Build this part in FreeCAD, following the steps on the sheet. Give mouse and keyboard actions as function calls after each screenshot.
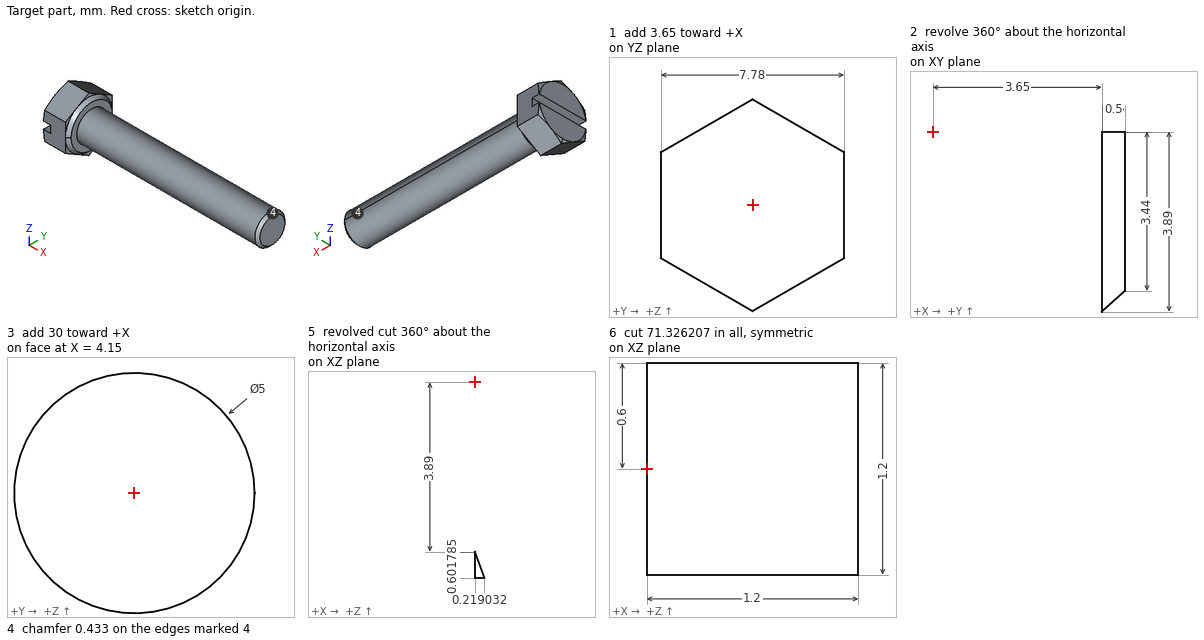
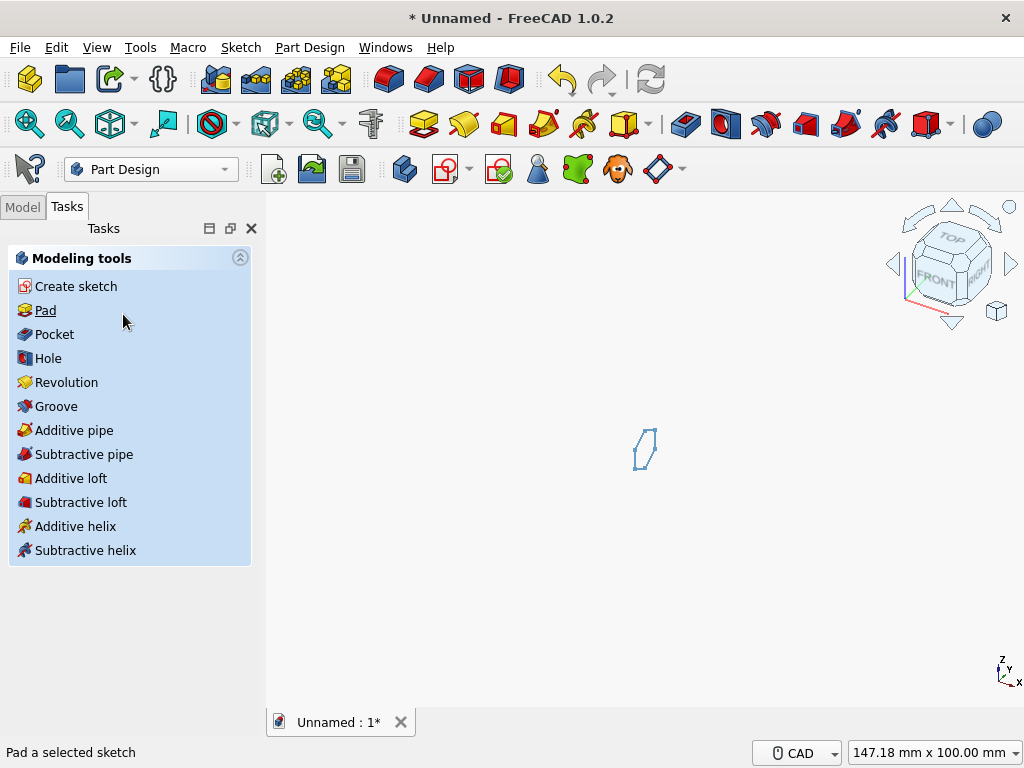
click(424, 124)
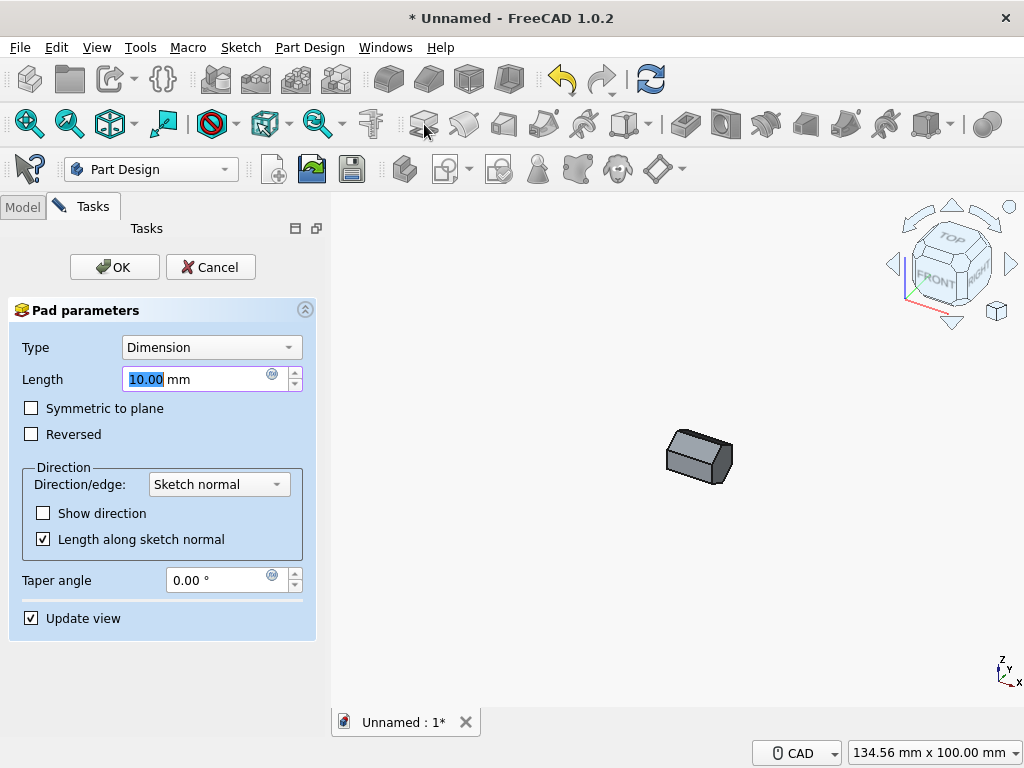
text(3.65)
key(Tab)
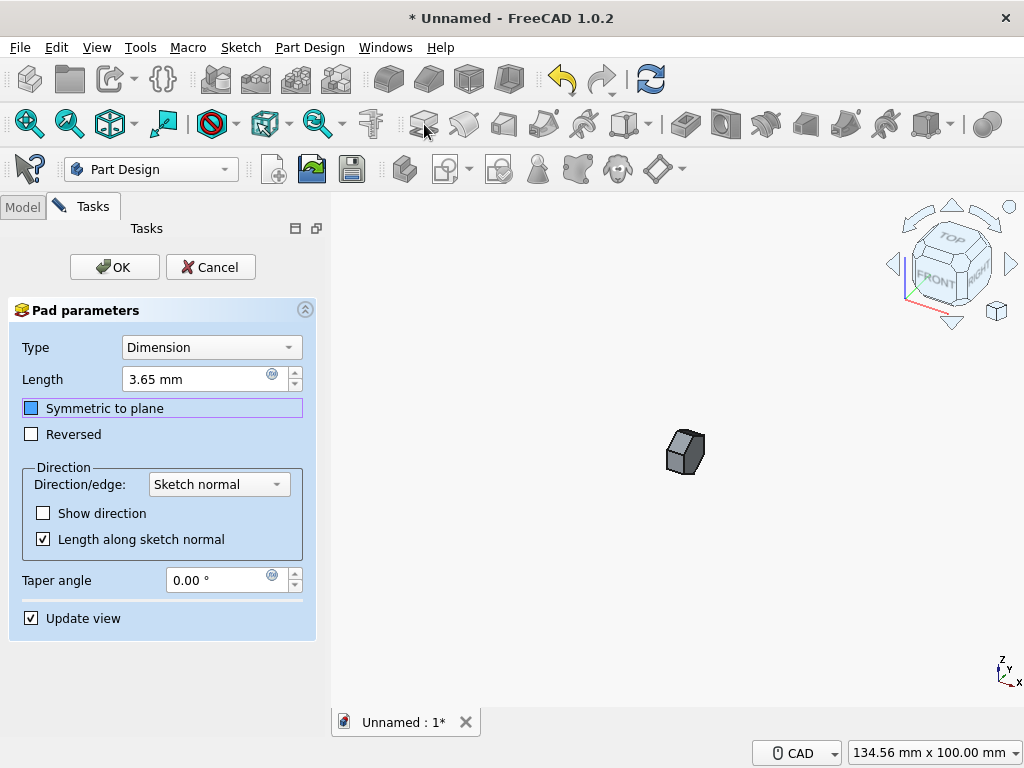
click(115, 267)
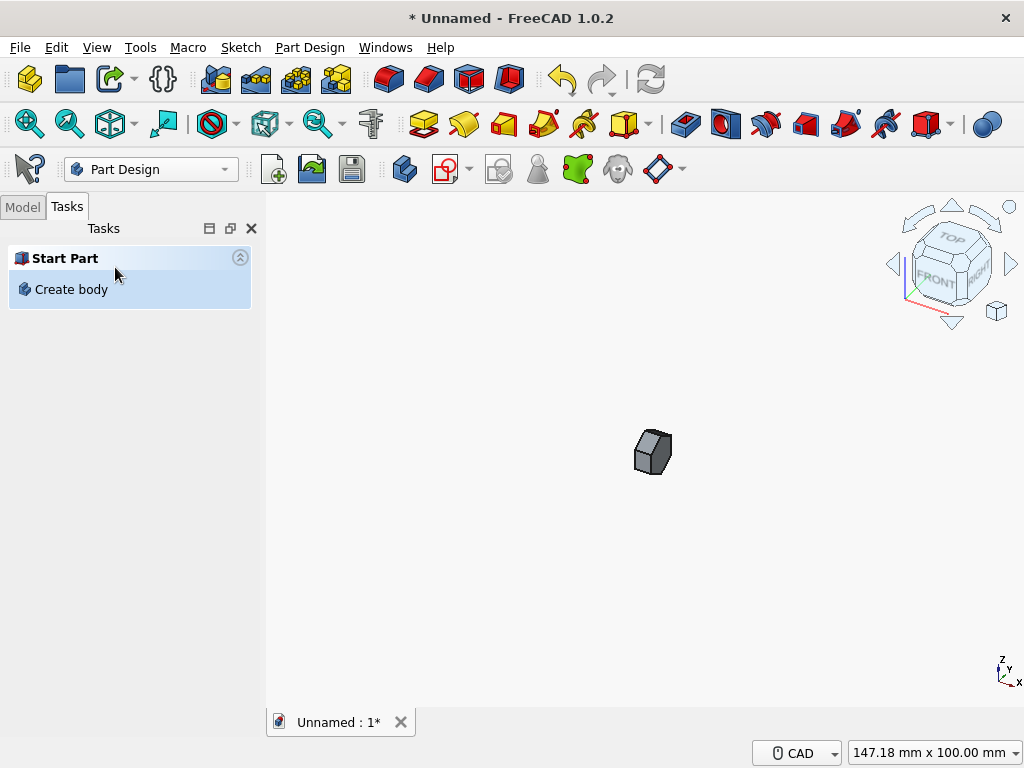
click(30, 124)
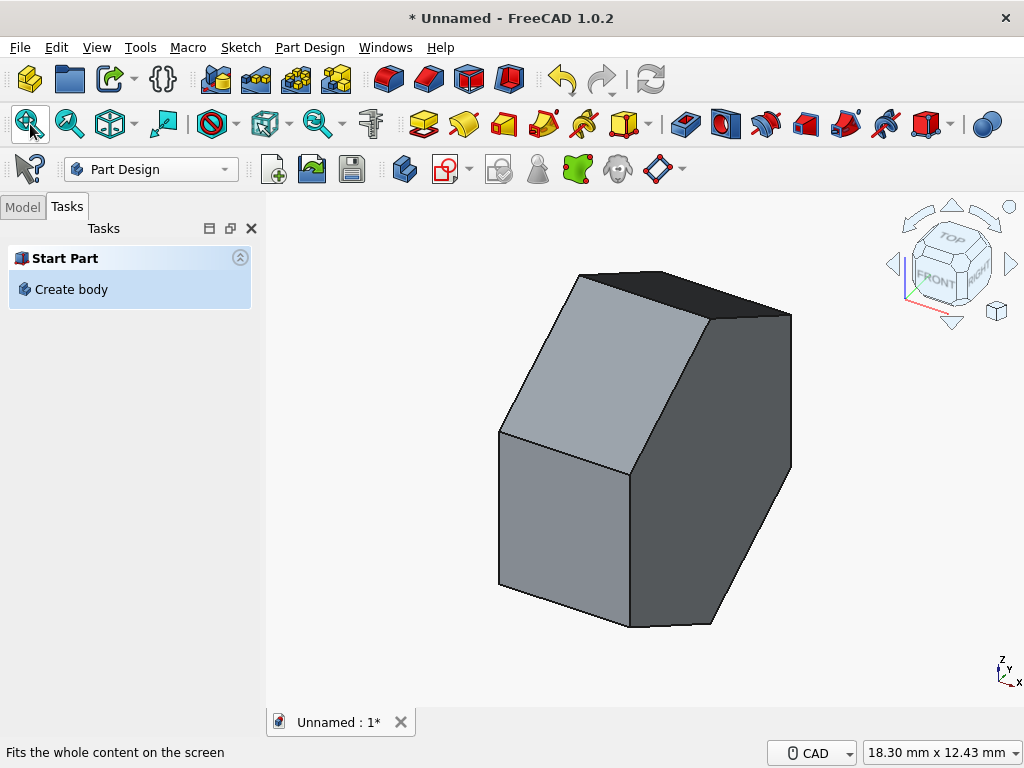
click(446, 170)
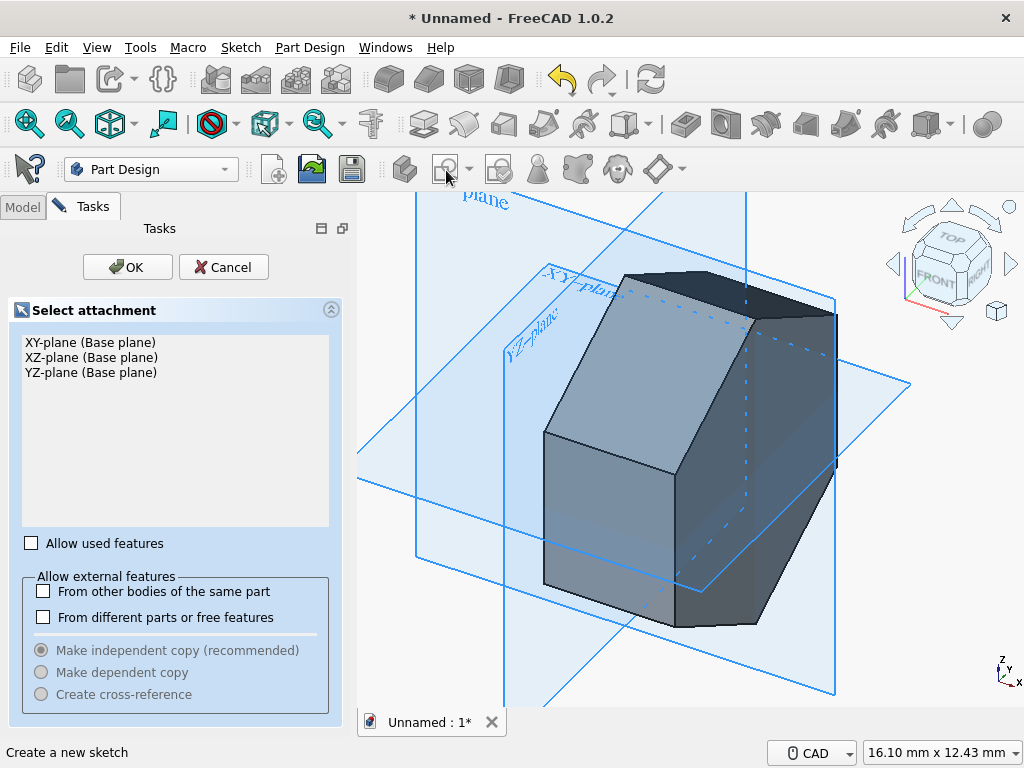
click(82, 342)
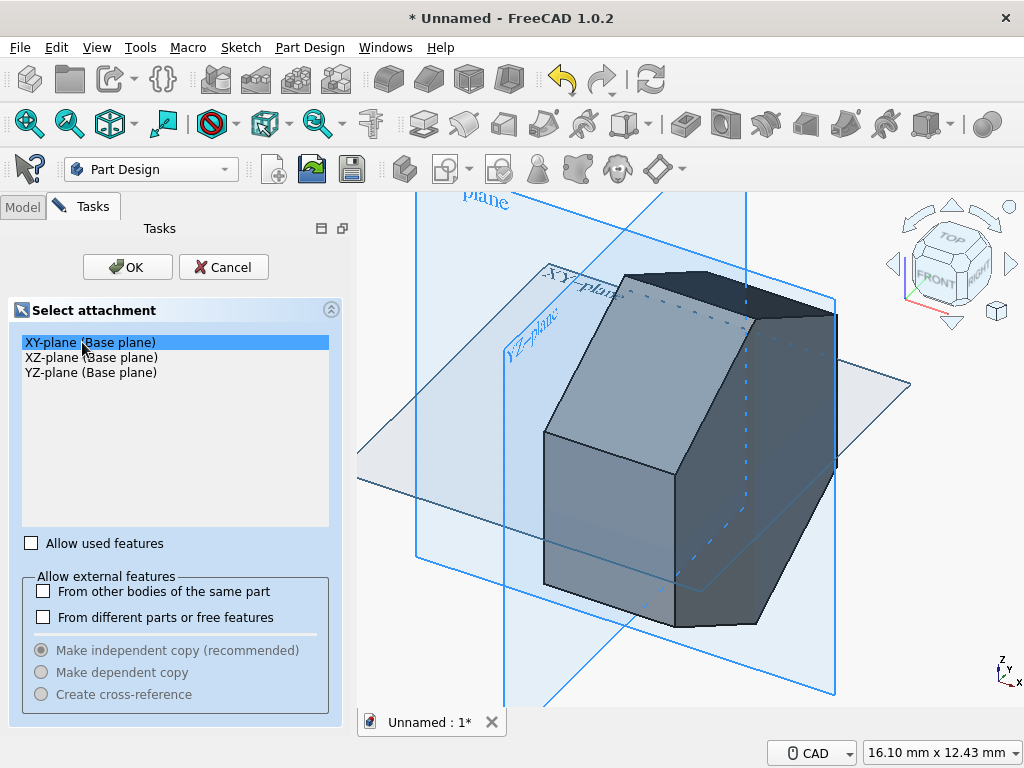
click(128, 267)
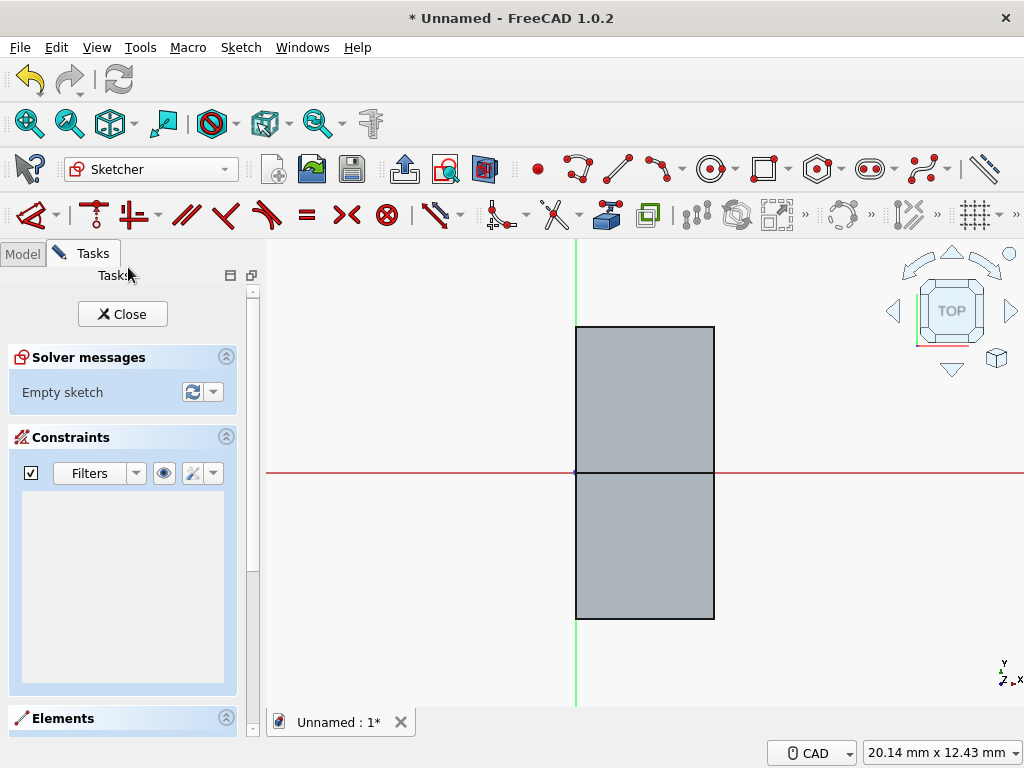
key(q)
key(s)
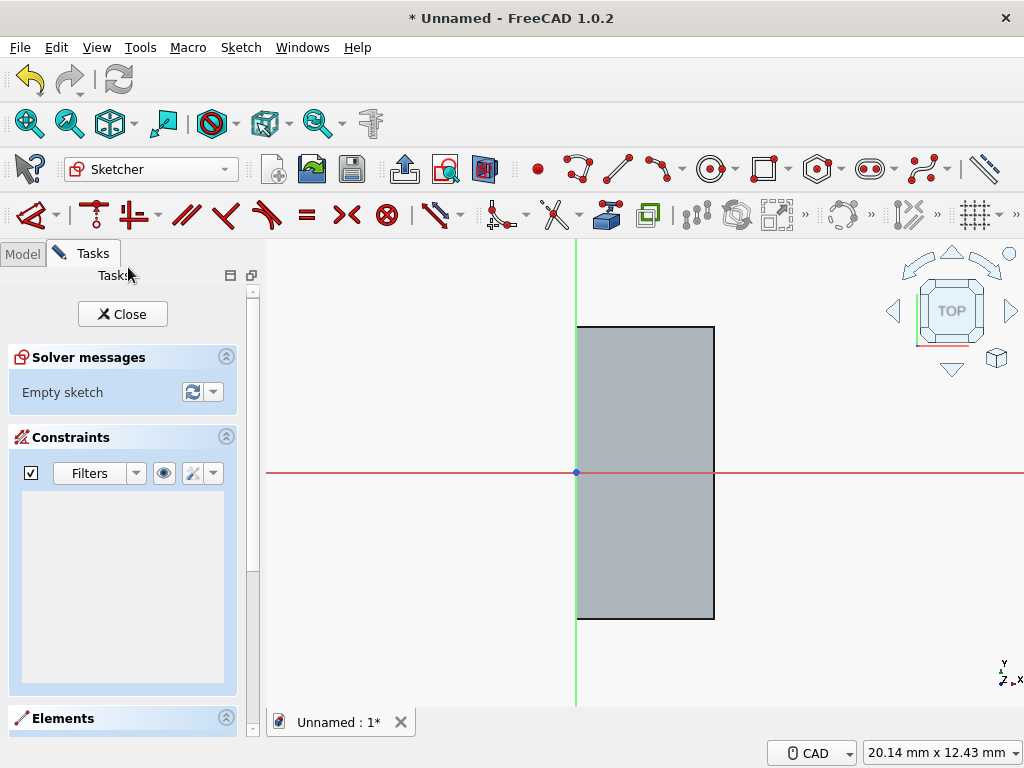
scroll(749, 635, up, 3)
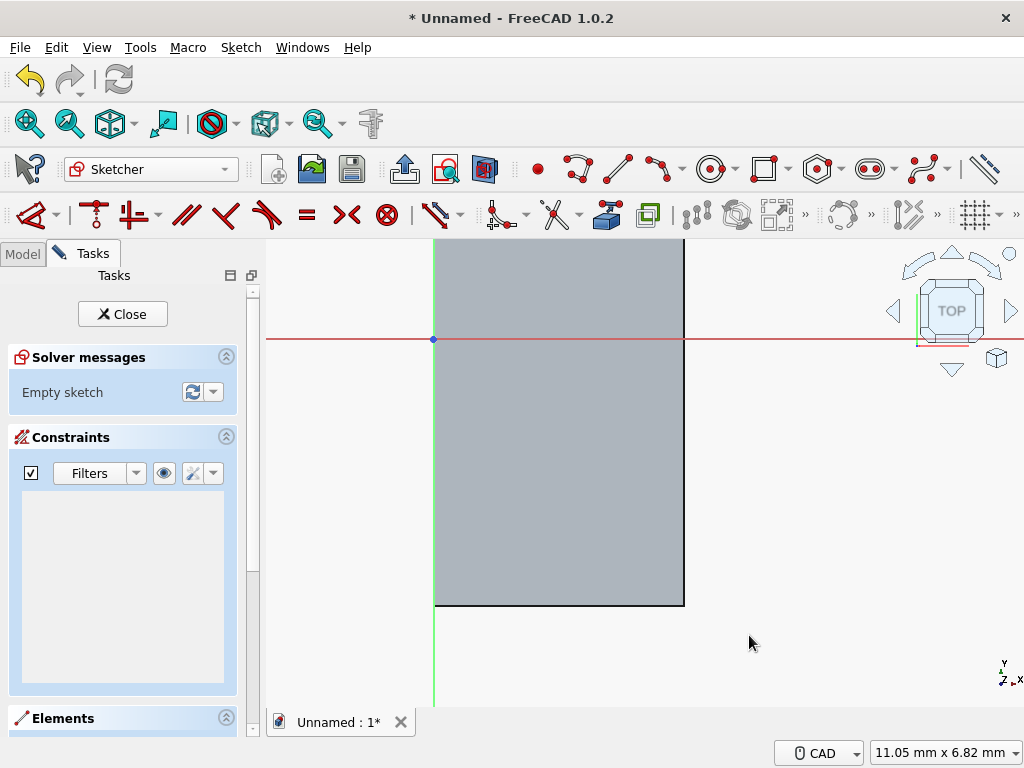
click(578, 170)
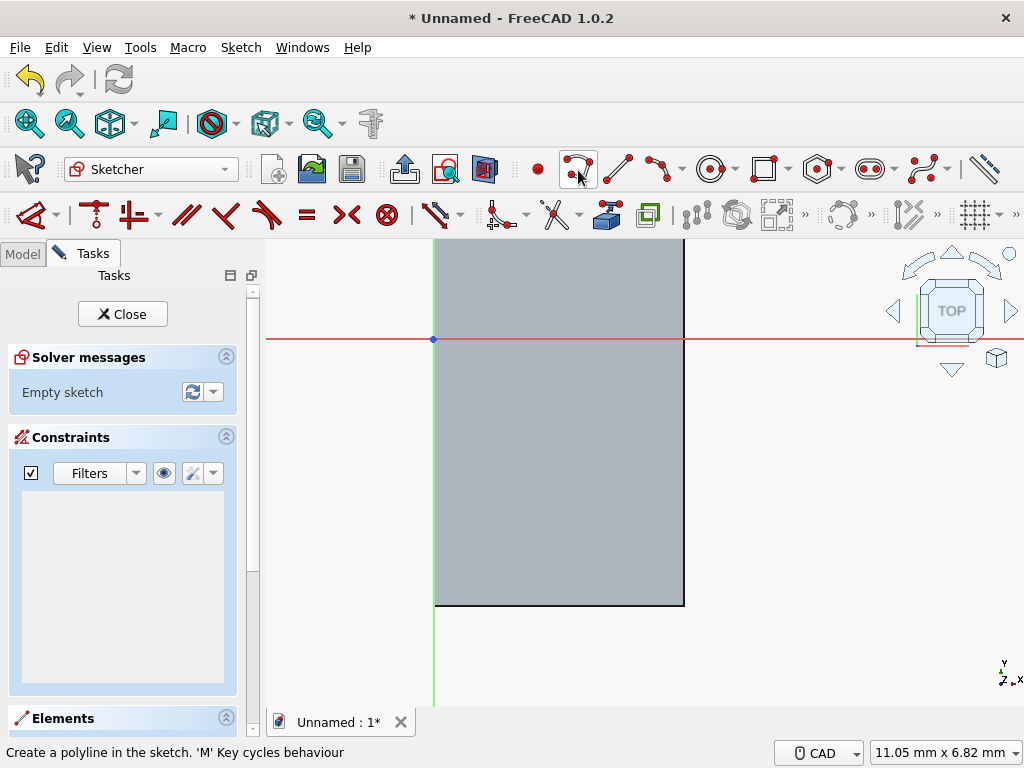
click(684, 339)
click(684, 606)
click(718, 575)
click(718, 348)
click(684, 339)
key(Escape)
key(Escape)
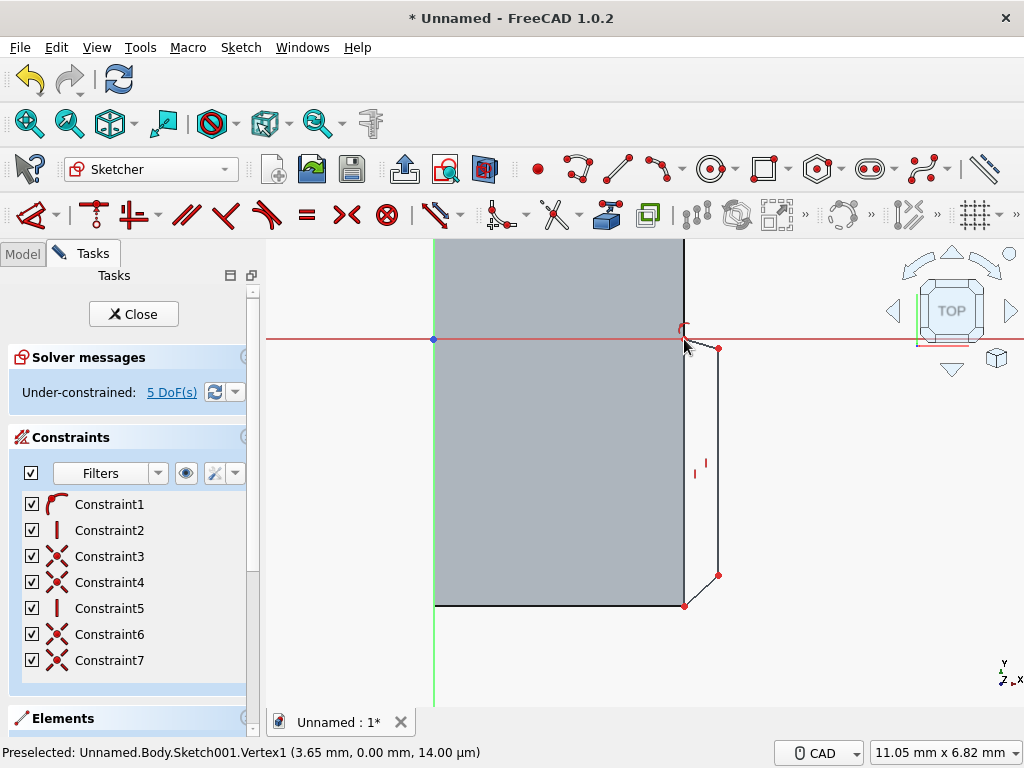
scroll(694, 342, up, 2)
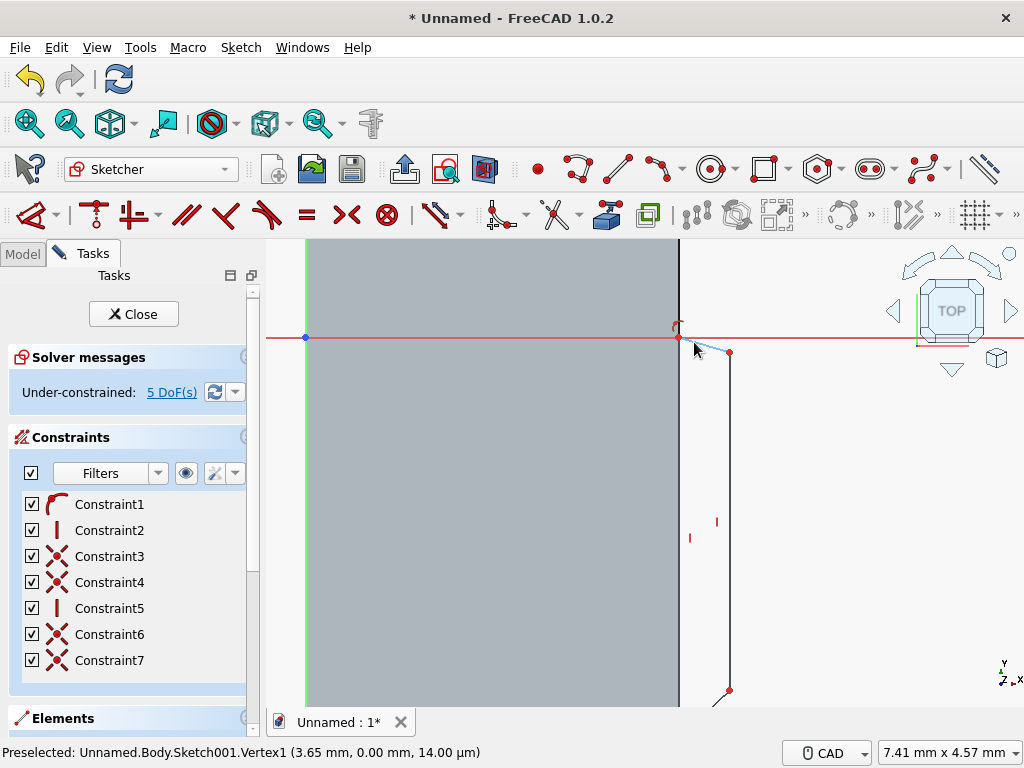
click(694, 342)